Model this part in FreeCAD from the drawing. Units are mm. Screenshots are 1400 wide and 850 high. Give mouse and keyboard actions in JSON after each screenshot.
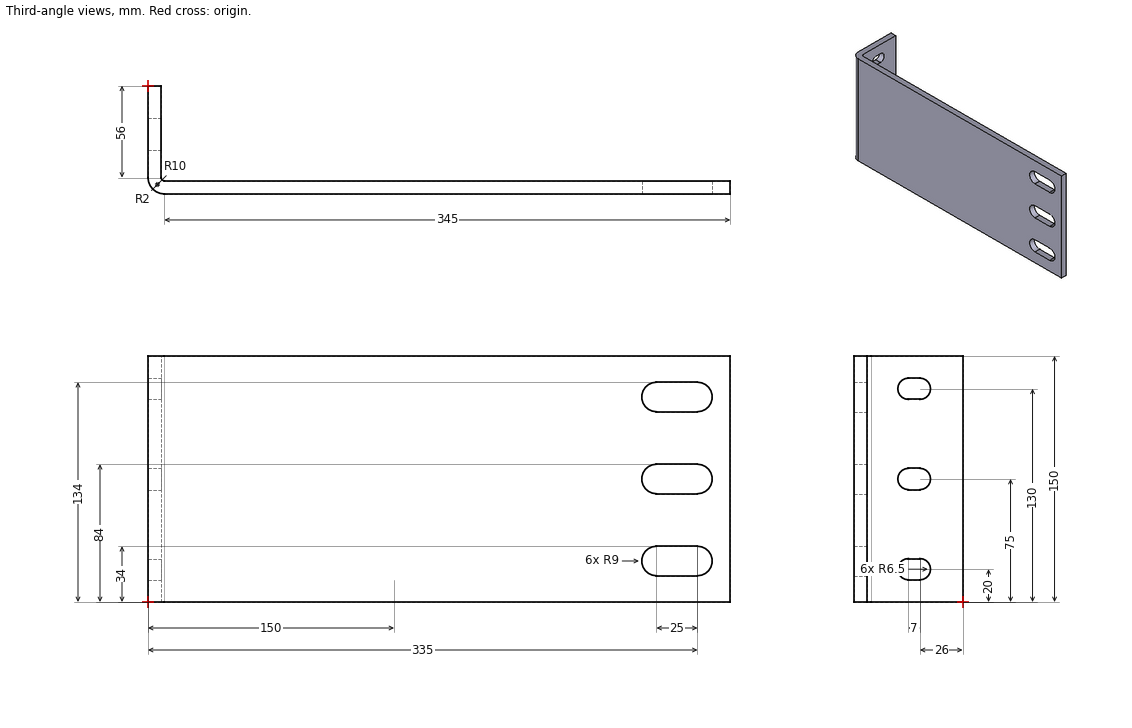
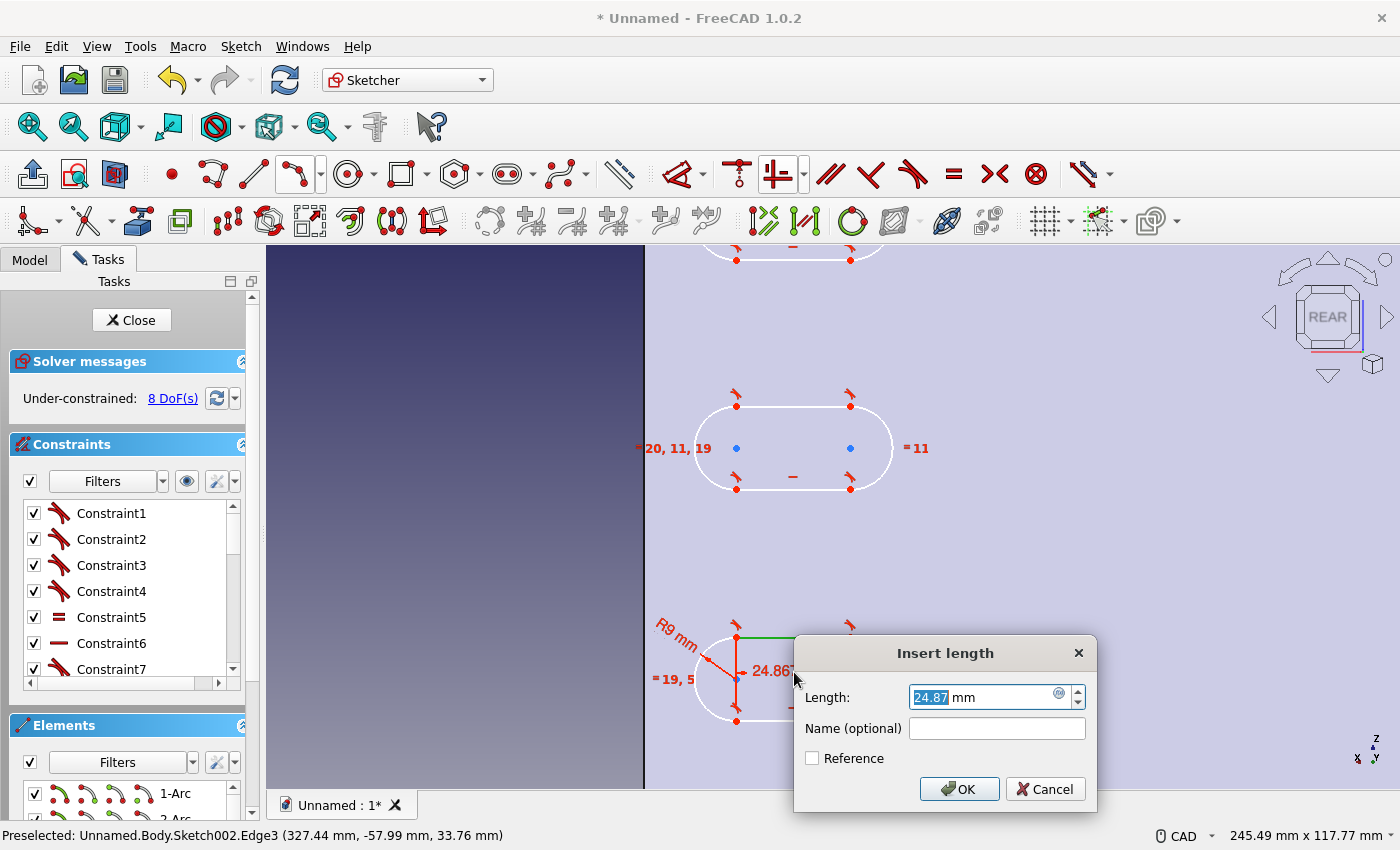
{"action": "type", "text": "25"}
{"action": "key", "text": "Return"}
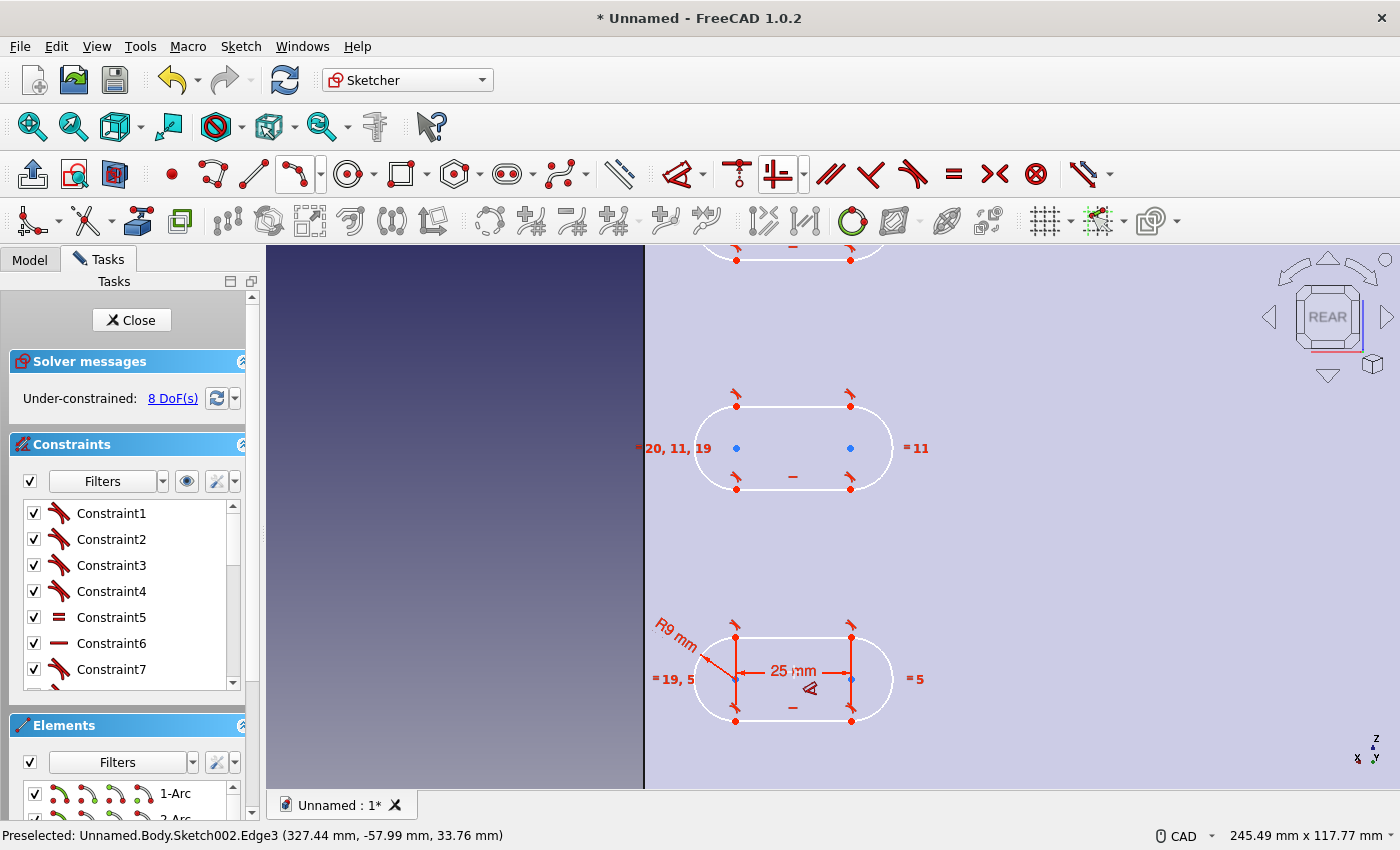
{"action": "left_click", "coordinate": [771, 407]}
{"action": "left_click", "coordinate": [794, 373]}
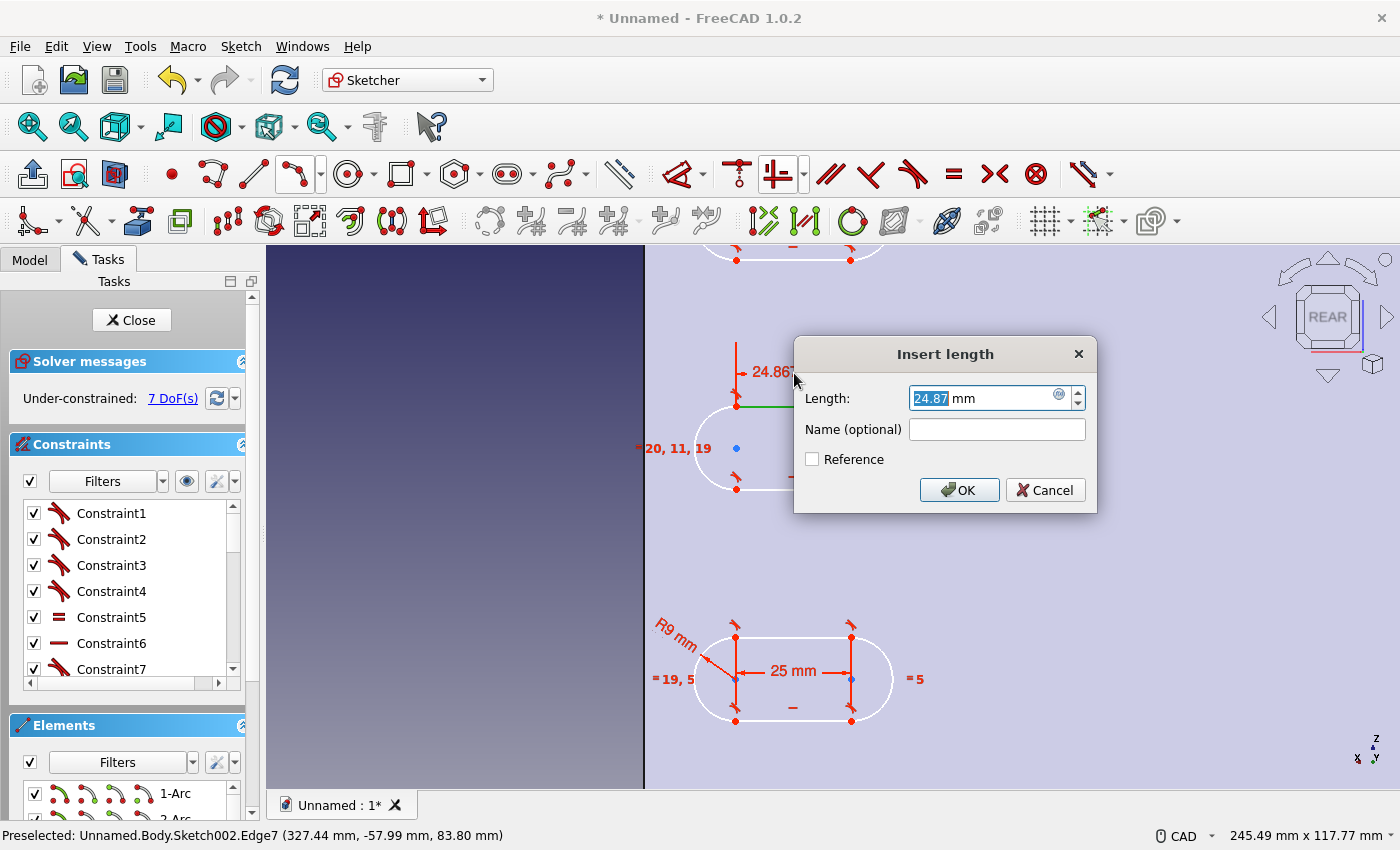
{"action": "type", "text": "25"}
{"action": "key", "text": "Return"}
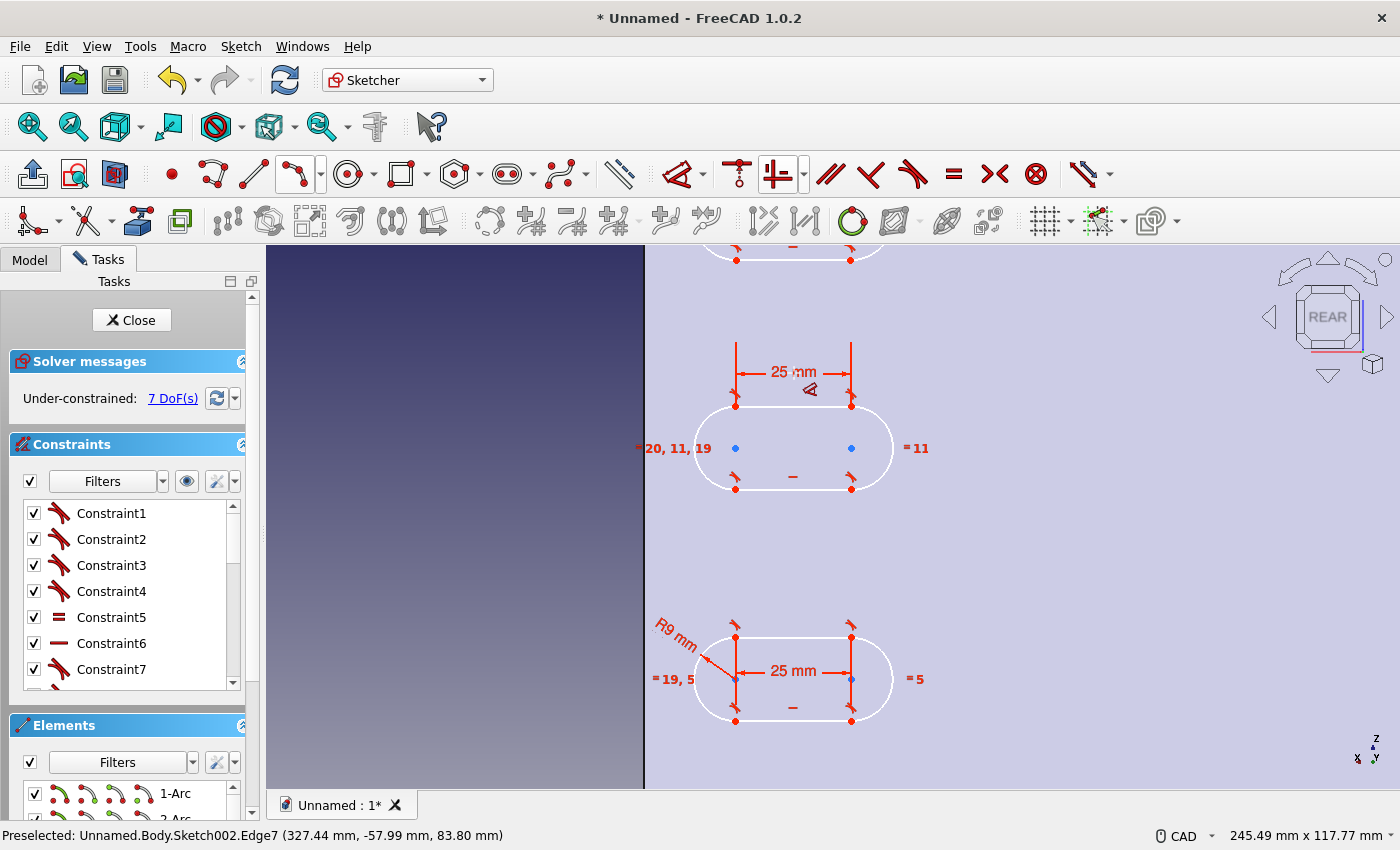
{"action": "scroll", "coordinate": [705, 659], "scroll_direction": "down", "scroll_amount": 2}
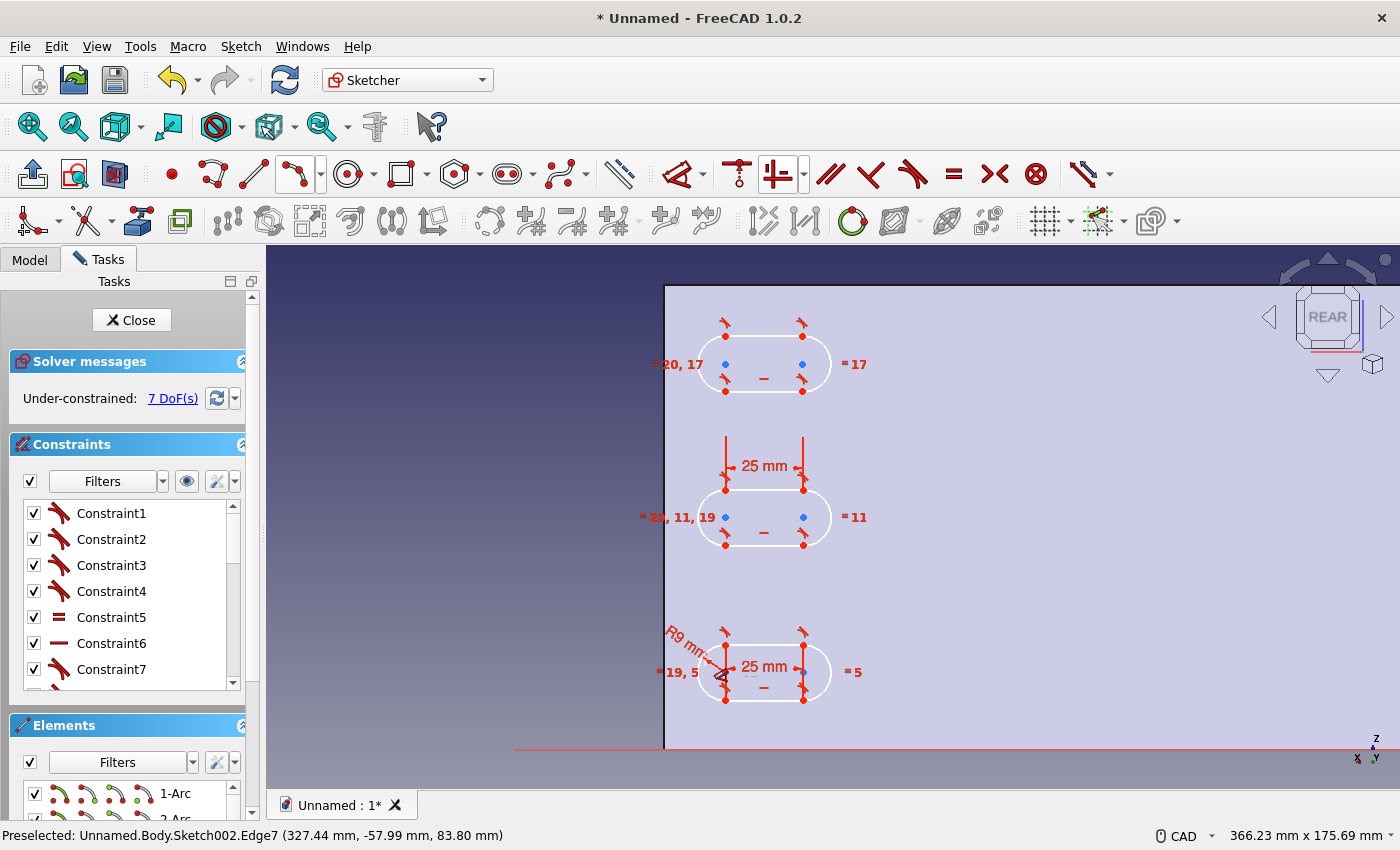
{"action": "left_click", "coordinate": [749, 336]}
{"action": "left_click", "coordinate": [764, 302]}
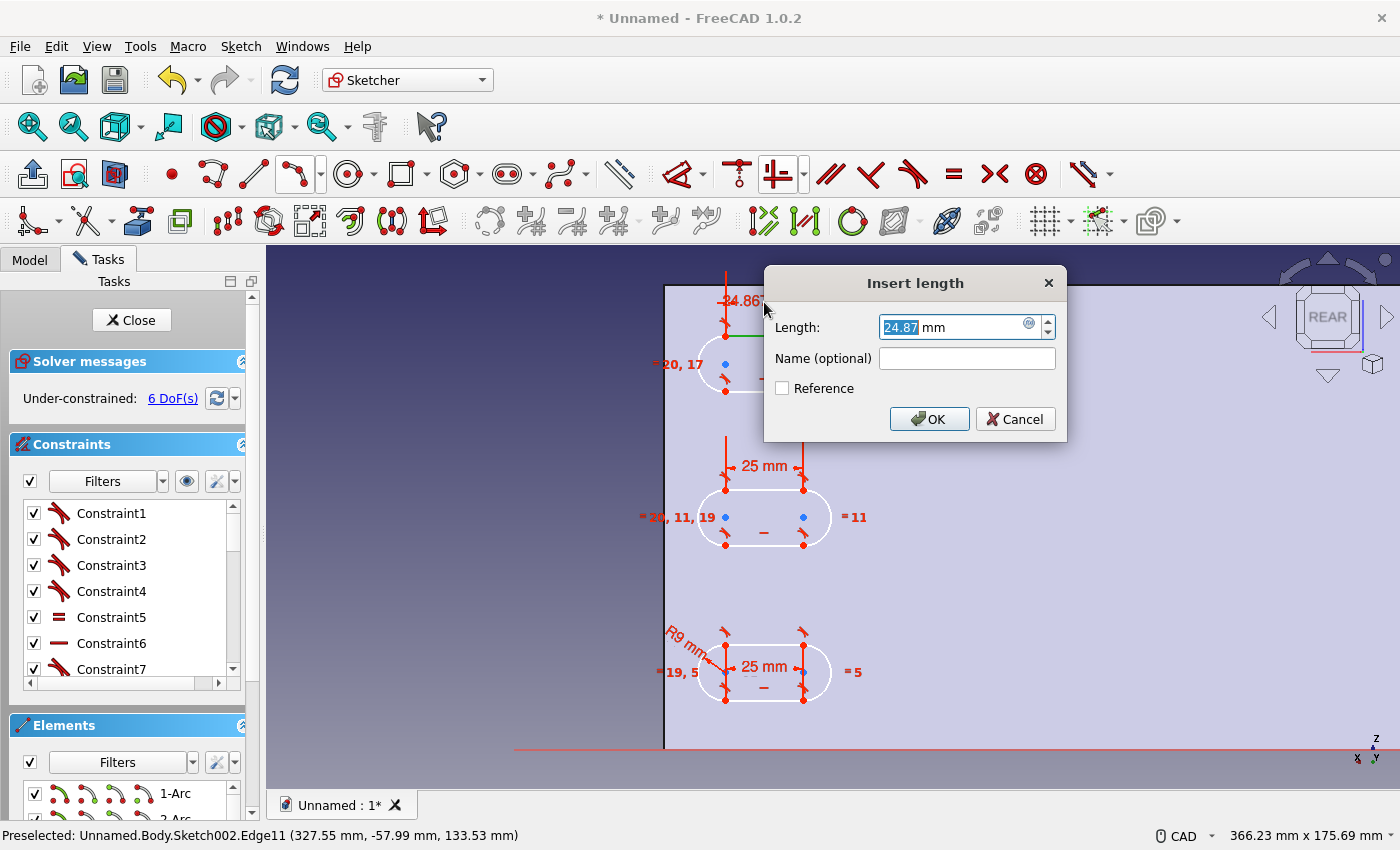
{"action": "type", "text": "25"}
{"action": "key", "text": "Return"}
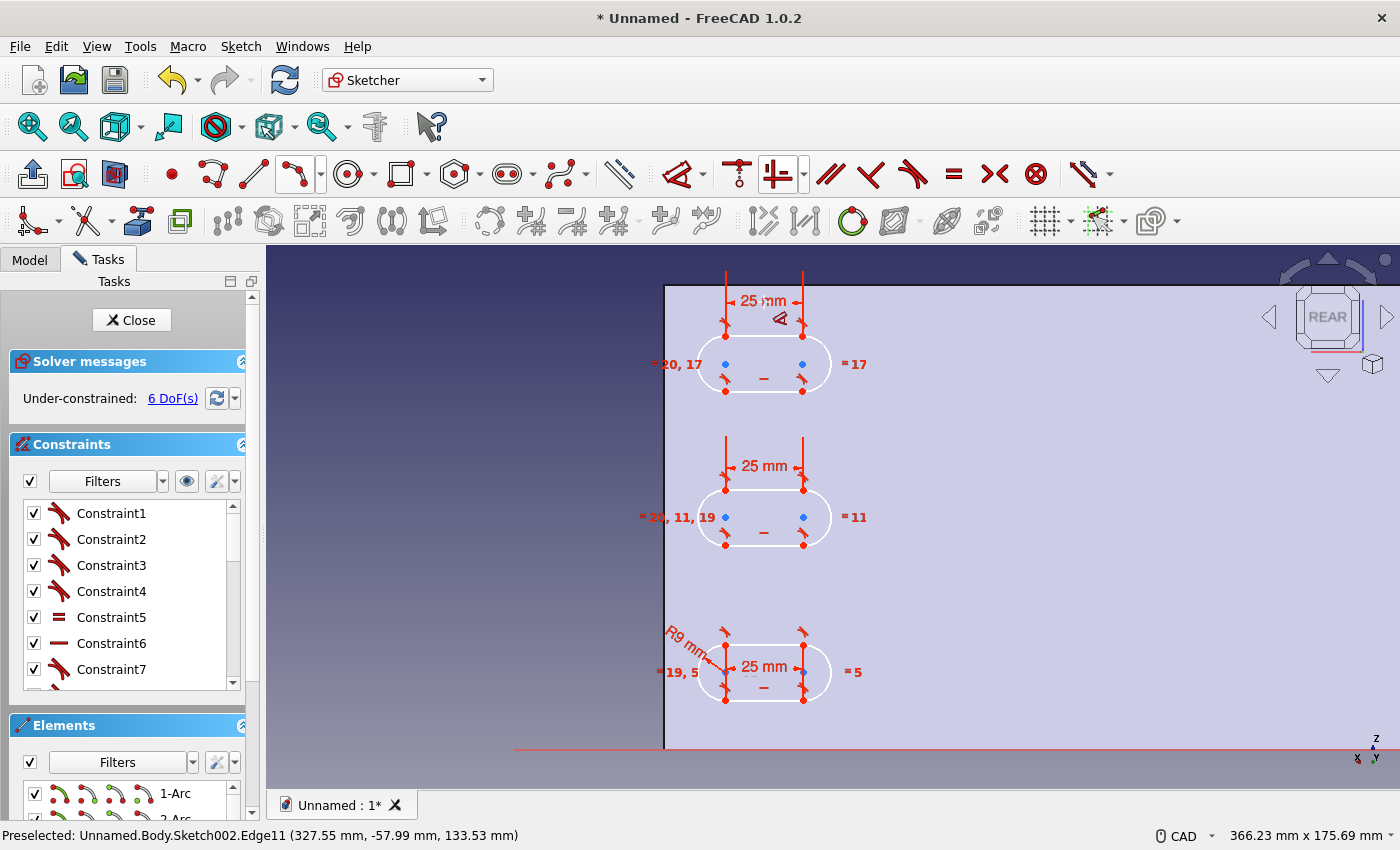
{"action": "left_click", "coordinate": [726, 645]}
{"action": "left_click", "coordinate": [692, 697]}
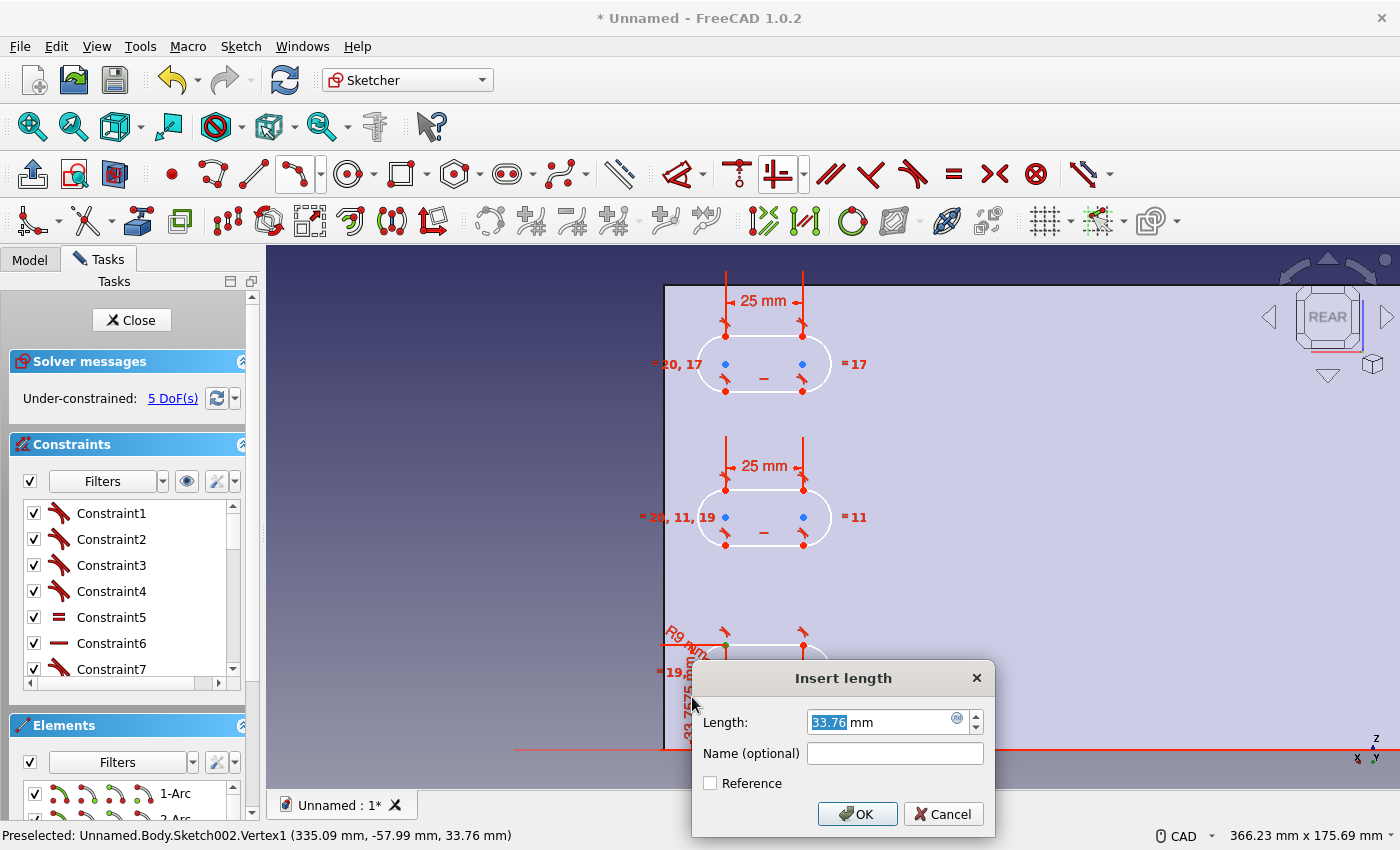
{"action": "type", "text": "34"}
{"action": "key", "text": "Return"}